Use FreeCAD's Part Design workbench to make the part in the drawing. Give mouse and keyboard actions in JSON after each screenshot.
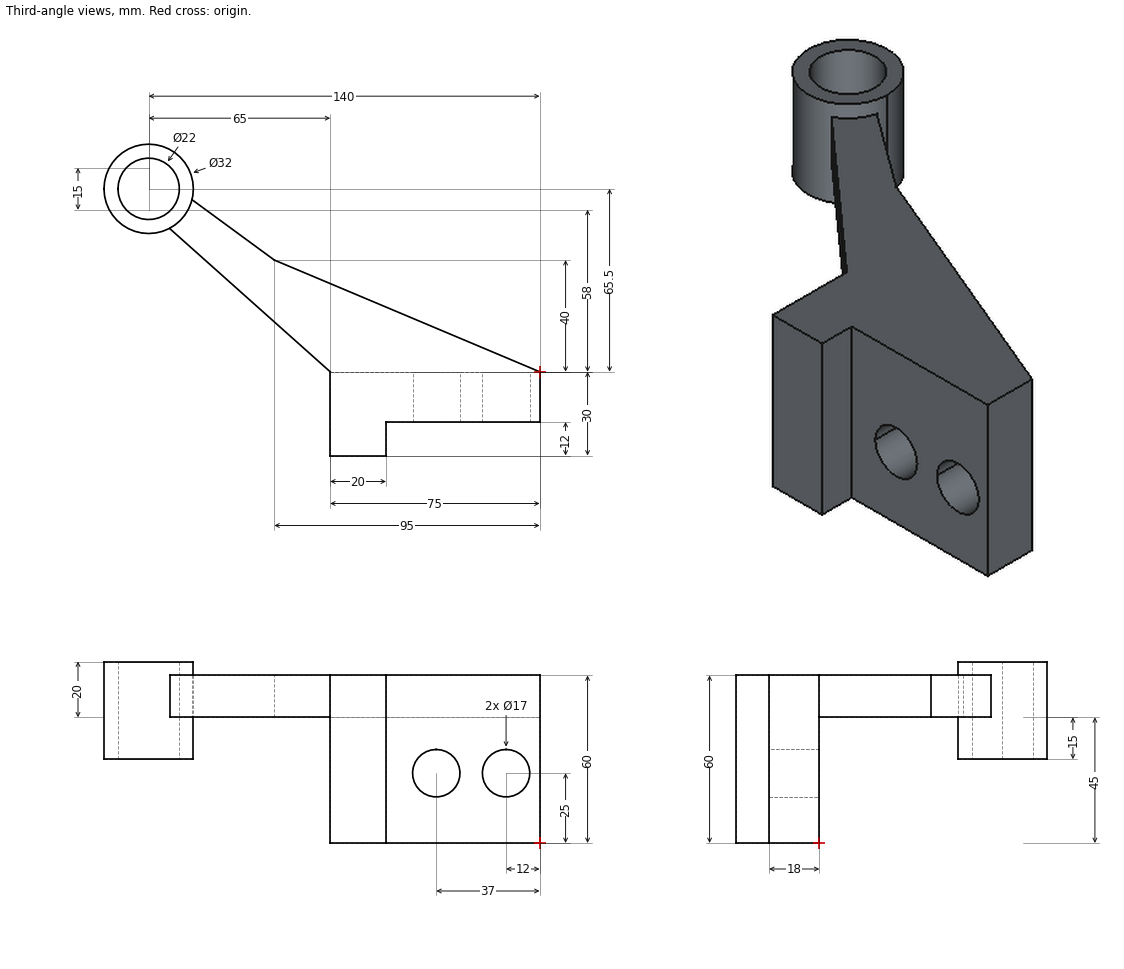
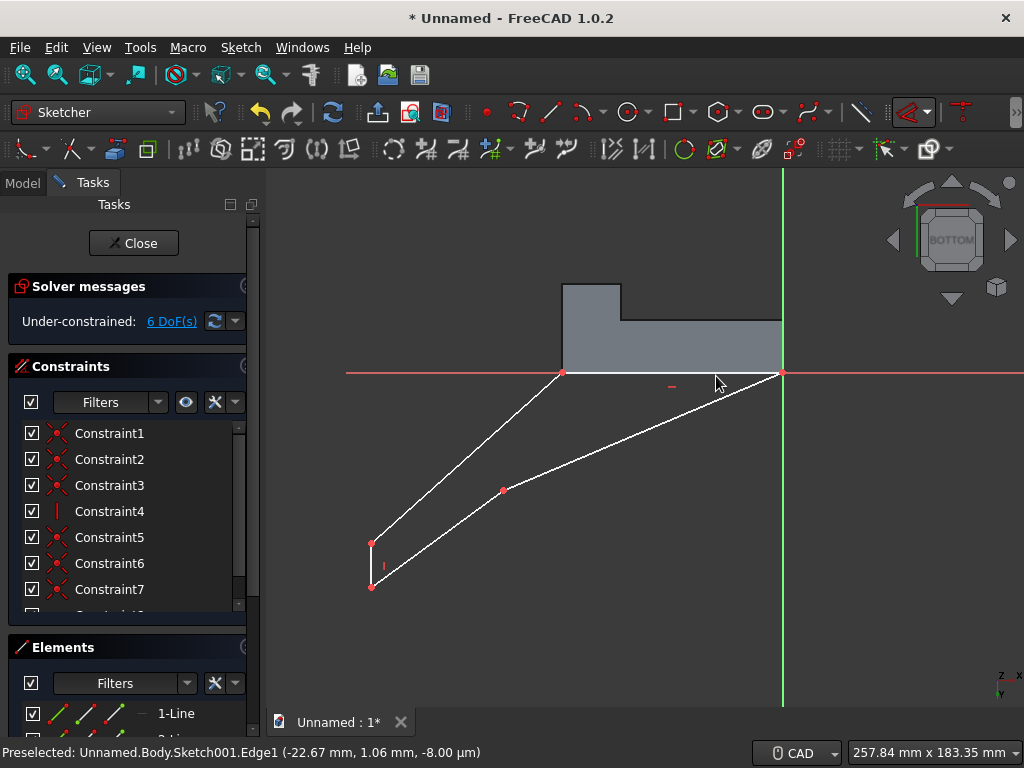
{"action": "left_click", "coordinate": [716, 373]}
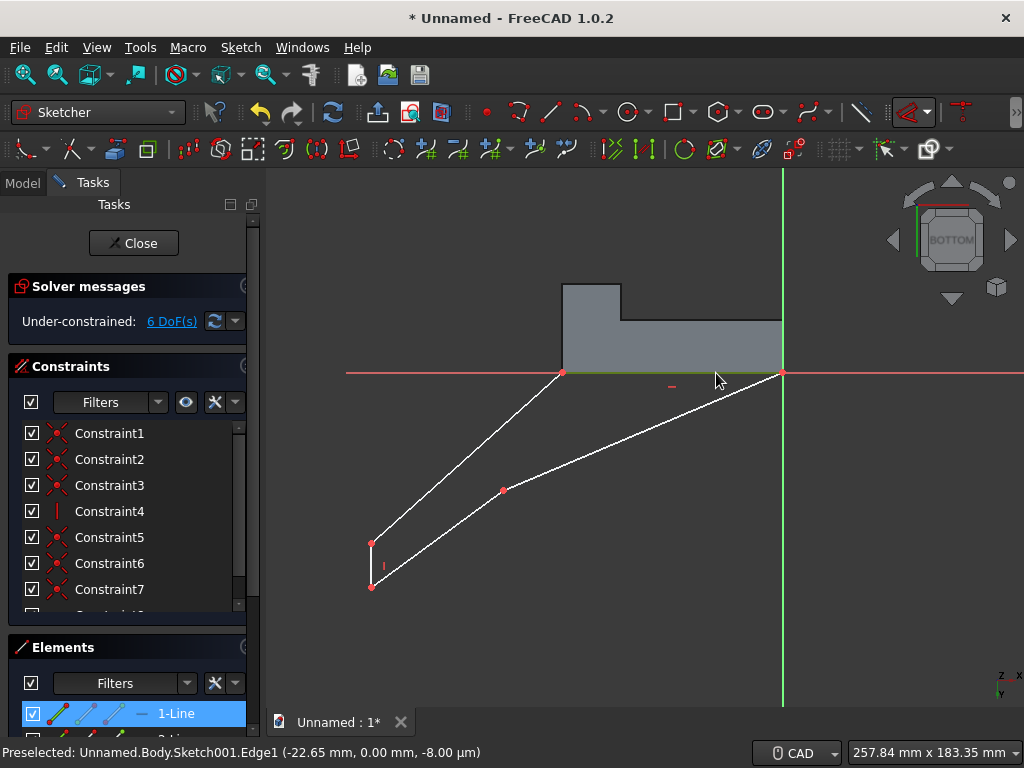
{"action": "key", "text": "l"}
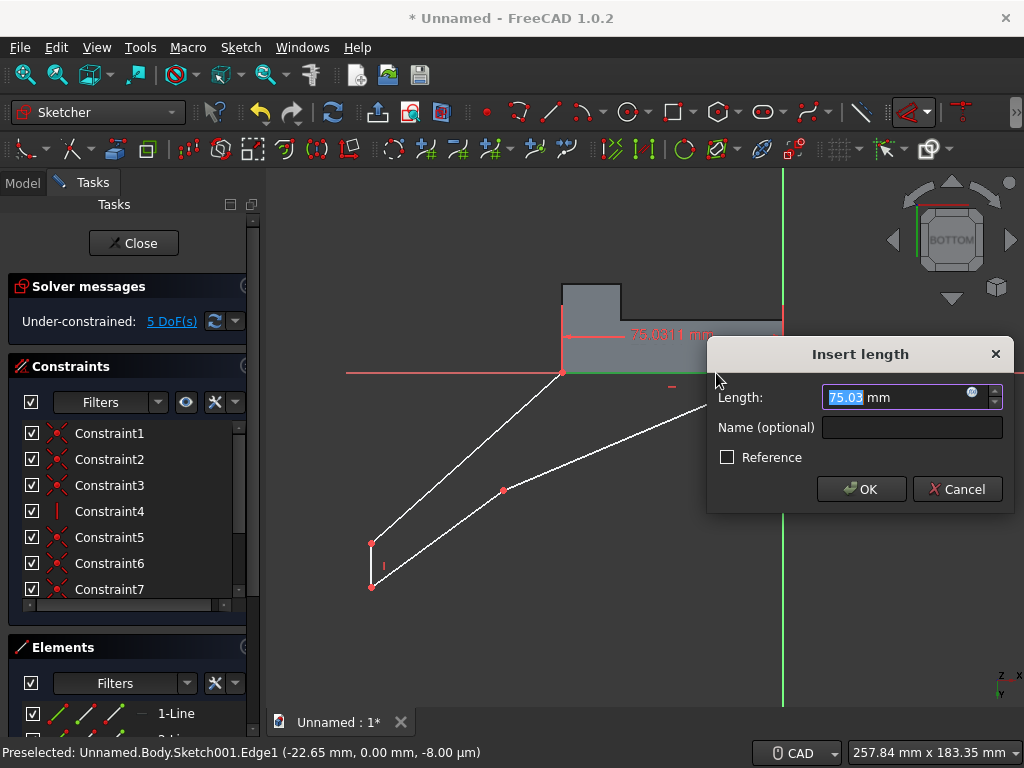
{"action": "type", "text": "75"}
{"action": "key", "text": "Return"}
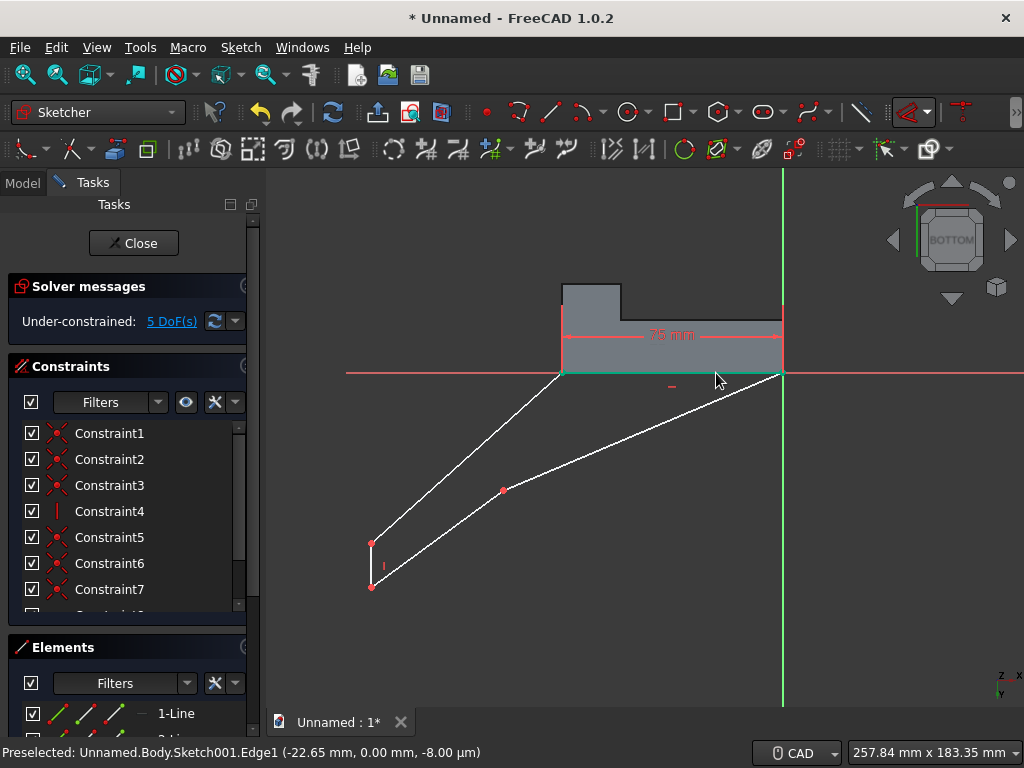
{"action": "left_click", "coordinate": [371, 557]}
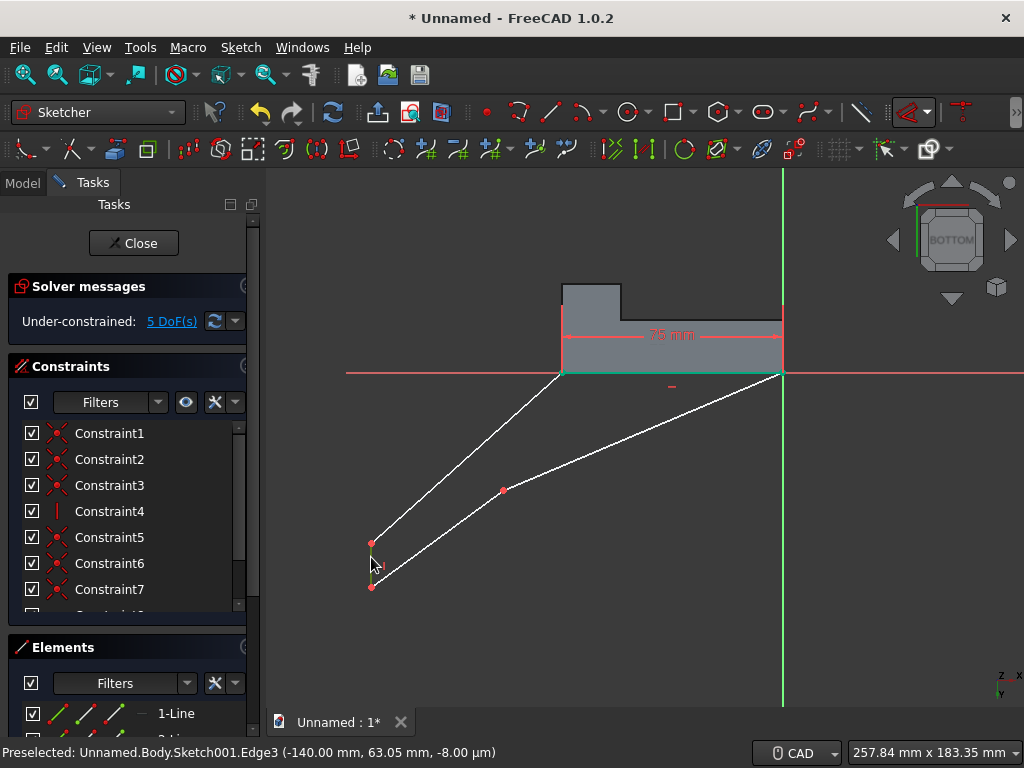
{"action": "left_click", "coordinate": [930, 112]}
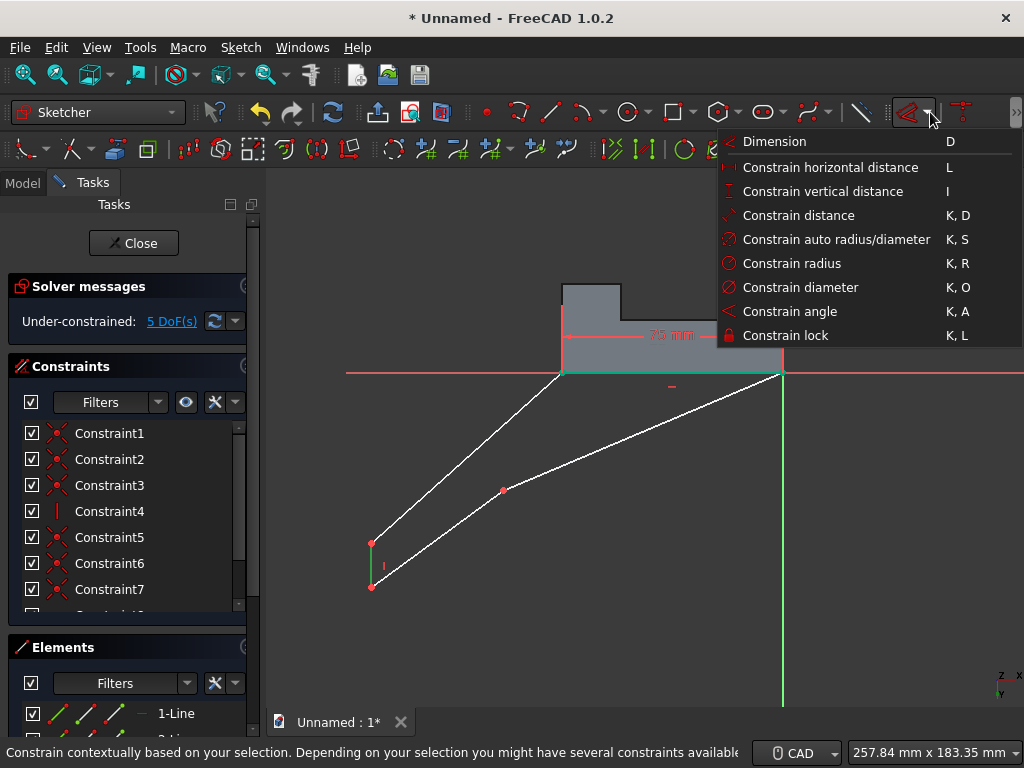
{"action": "left_click", "coordinate": [870, 191]}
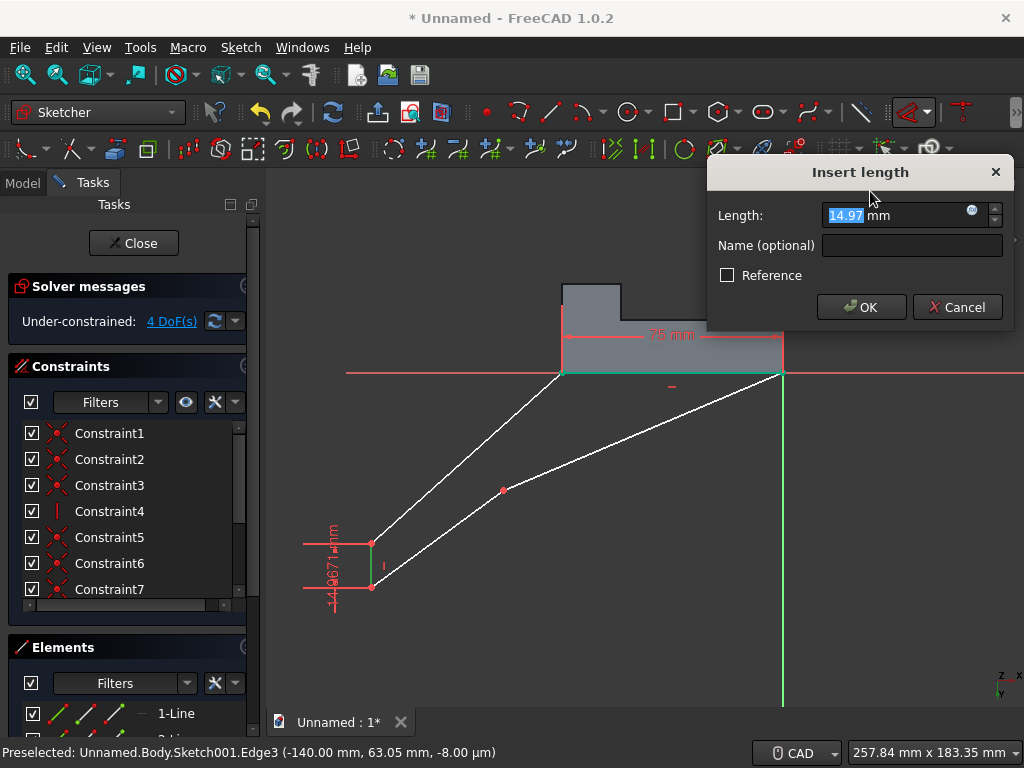
{"action": "type", "text": "15"}
{"action": "key", "text": "Return"}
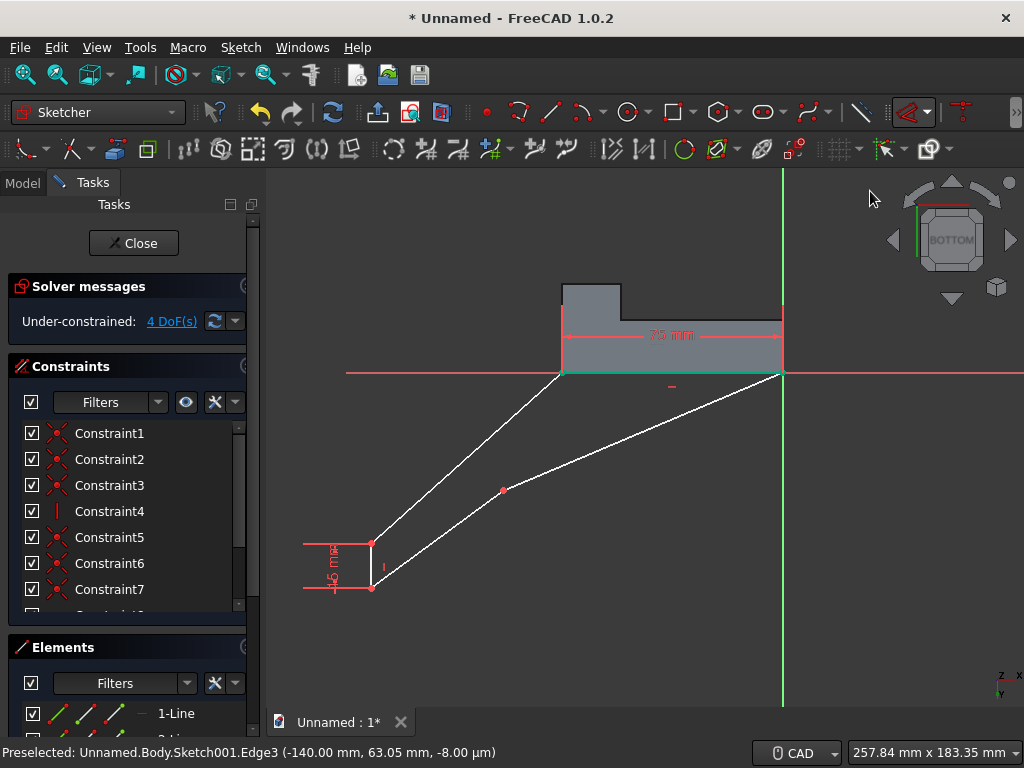
{"action": "left_click", "coordinate": [371, 544]}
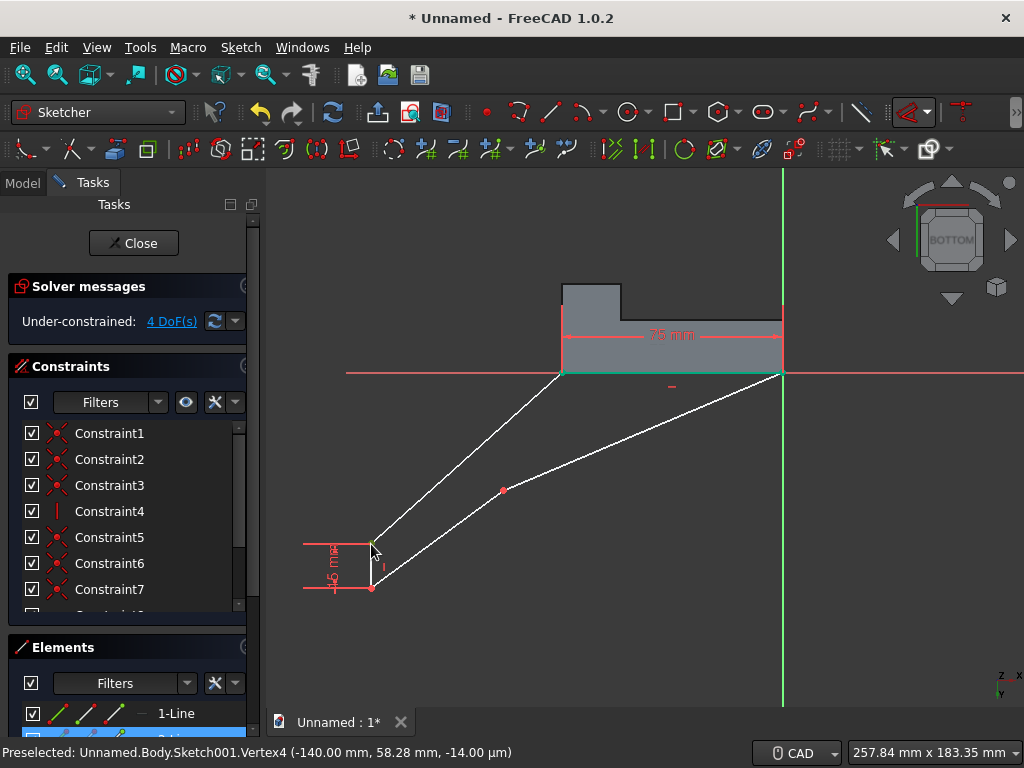
{"action": "left_click", "coordinate": [930, 112]}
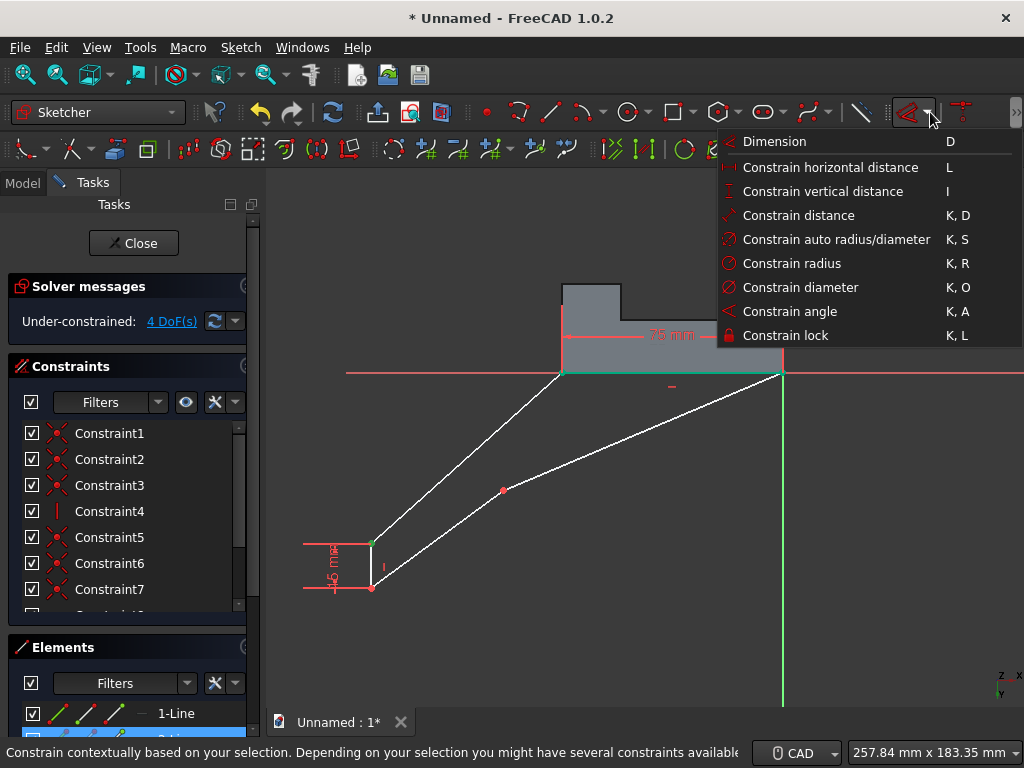
{"action": "left_click", "coordinate": [870, 191]}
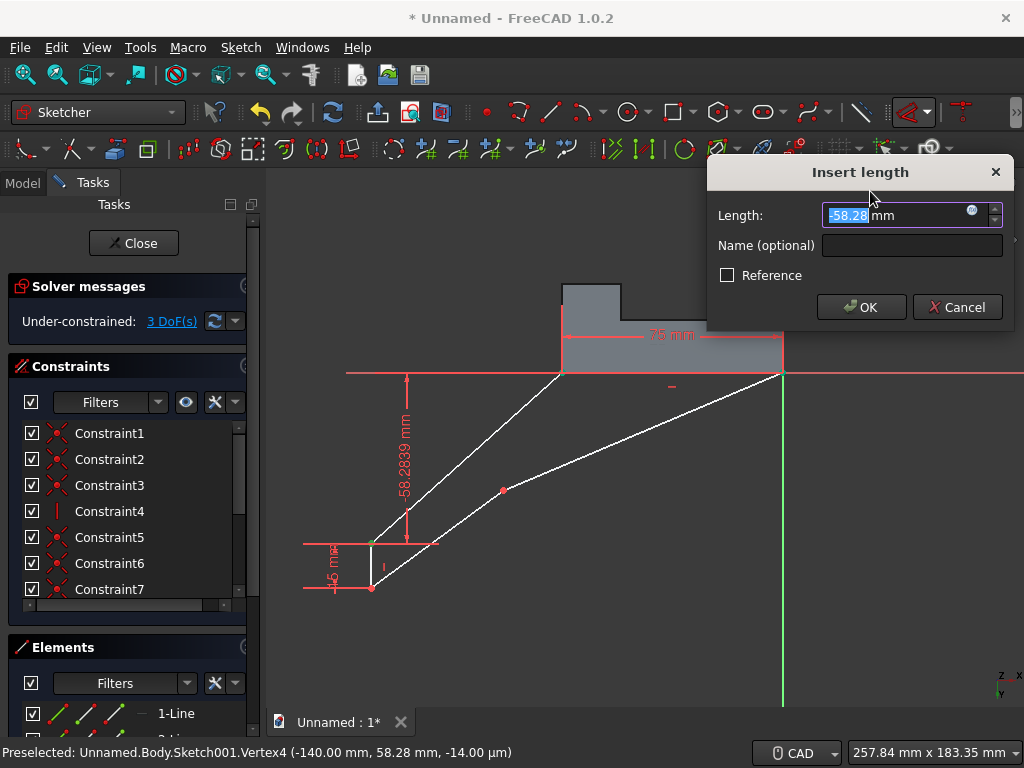
{"action": "type", "text": "-58"}
{"action": "key", "text": "Return"}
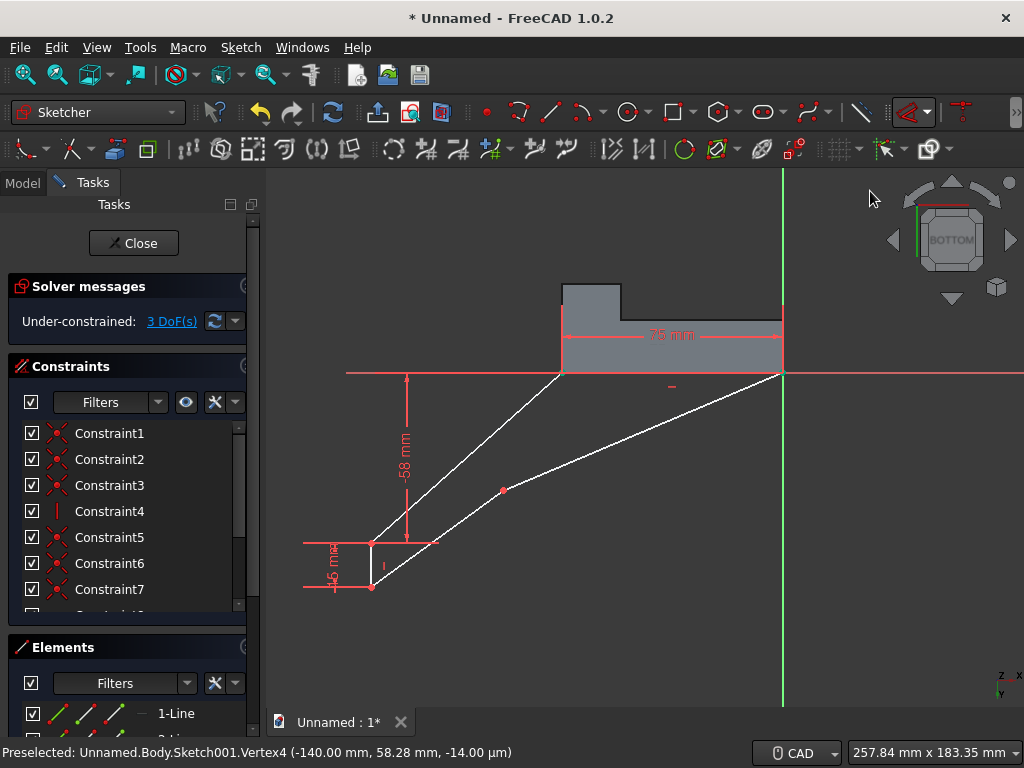
{"action": "left_click", "coordinate": [503, 491]}